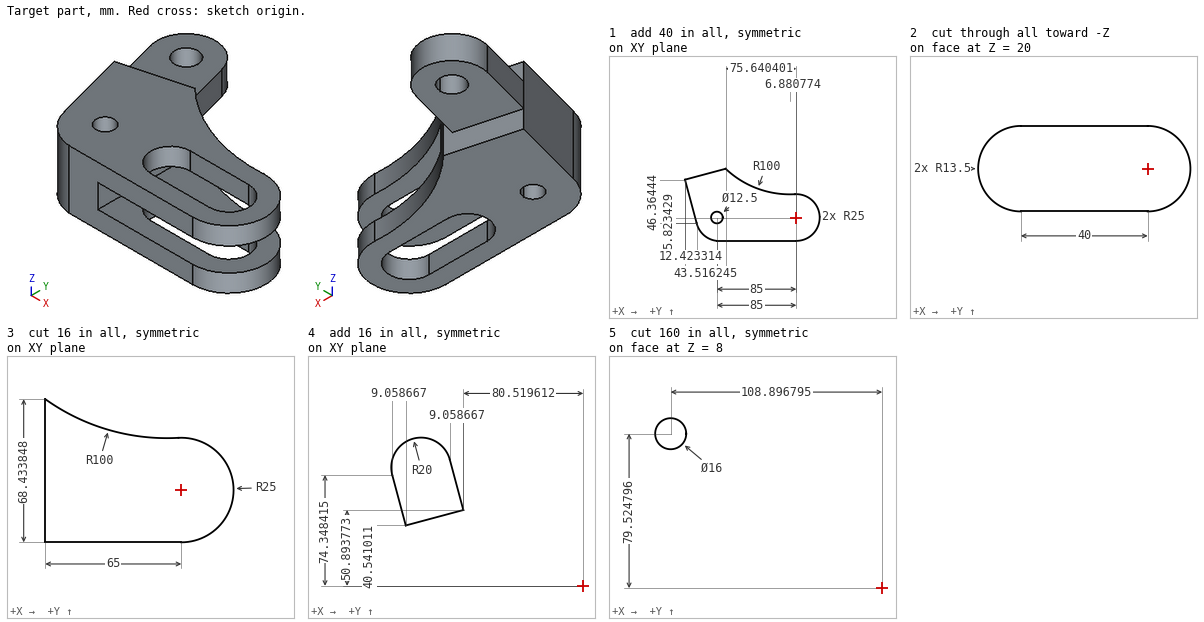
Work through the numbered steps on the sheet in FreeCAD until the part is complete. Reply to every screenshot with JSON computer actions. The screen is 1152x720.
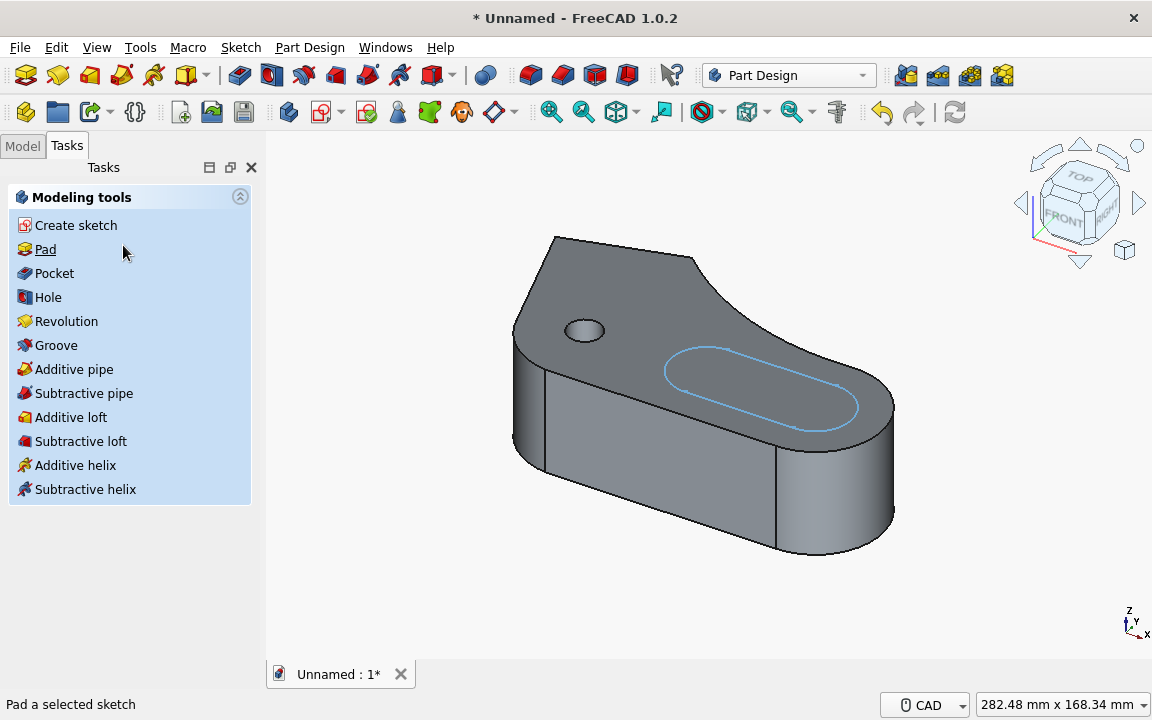
{"action": "left_click", "coordinate": [240, 76]}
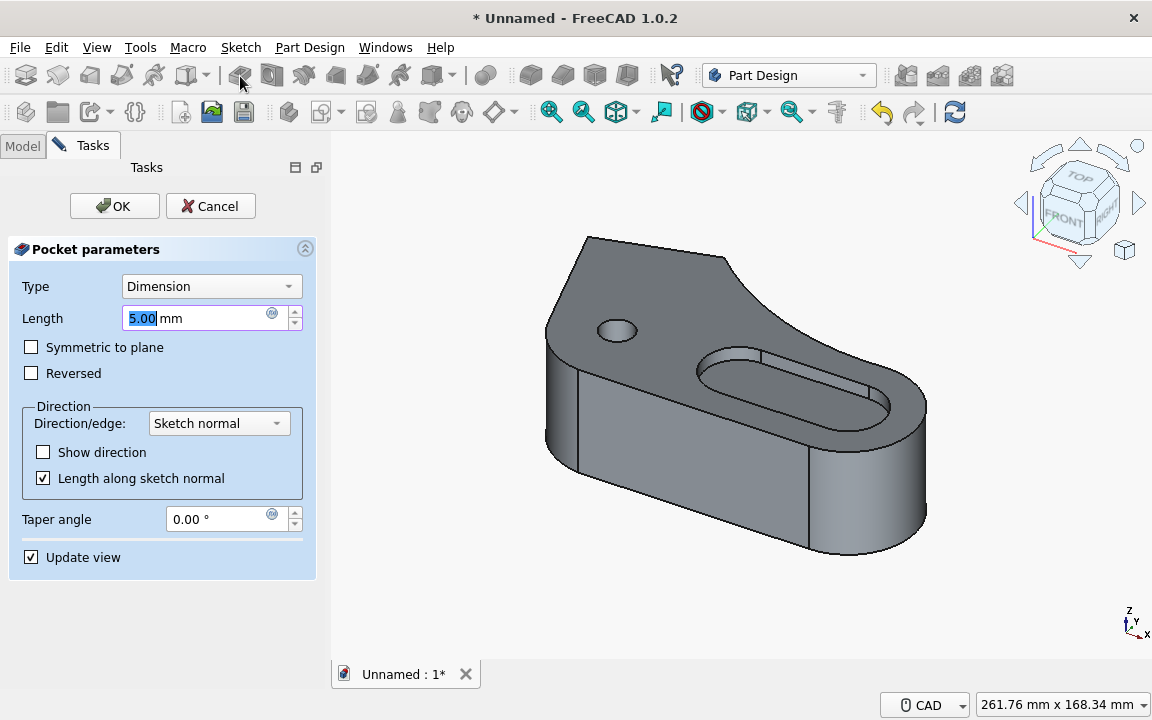
{"action": "left_click", "coordinate": [212, 286]}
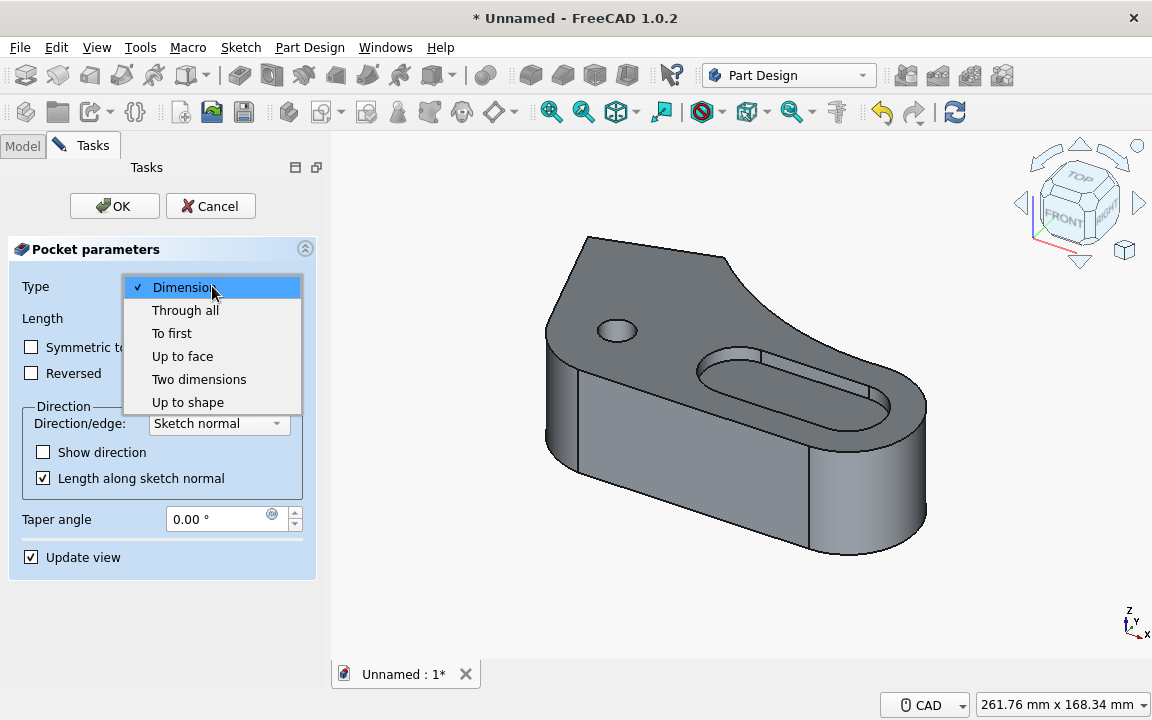
{"action": "left_click", "coordinate": [212, 310]}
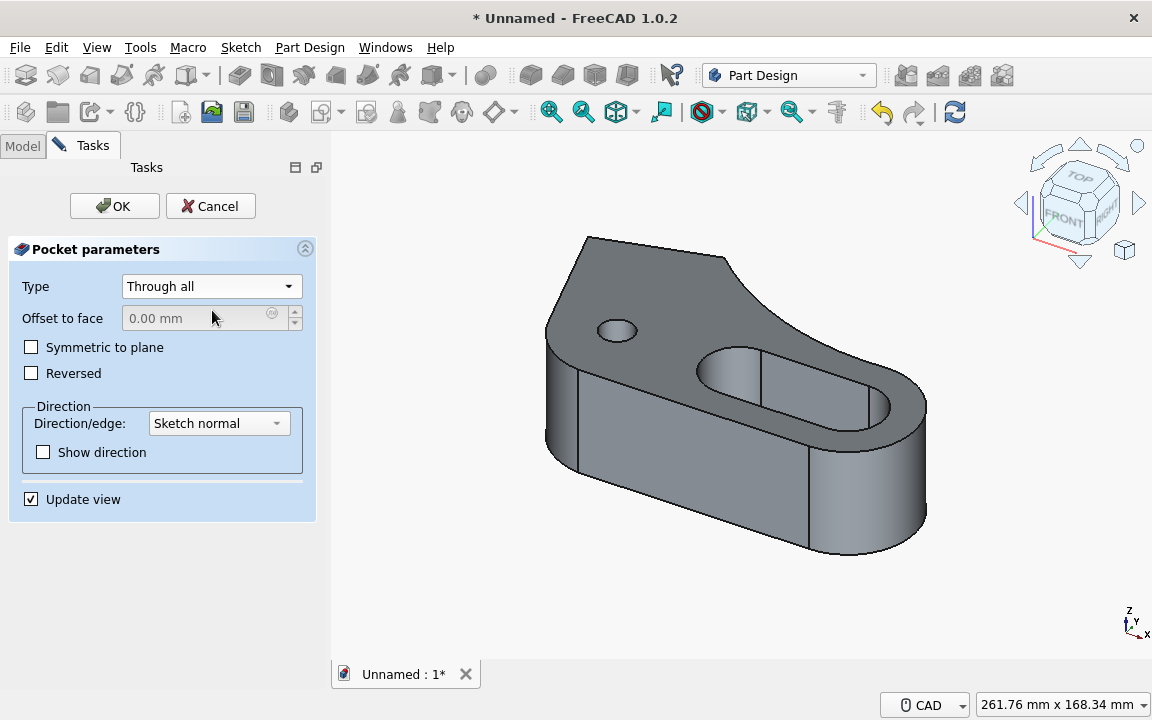
{"action": "left_click", "coordinate": [115, 206]}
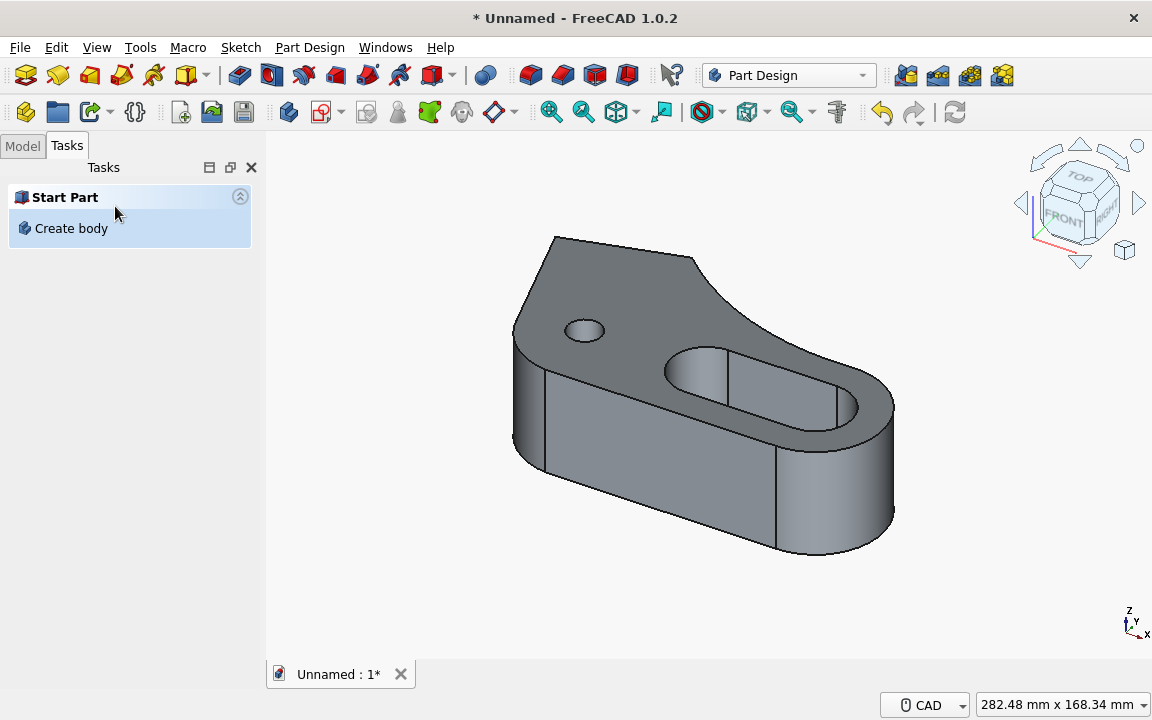
{"action": "left_click", "coordinate": [322, 112]}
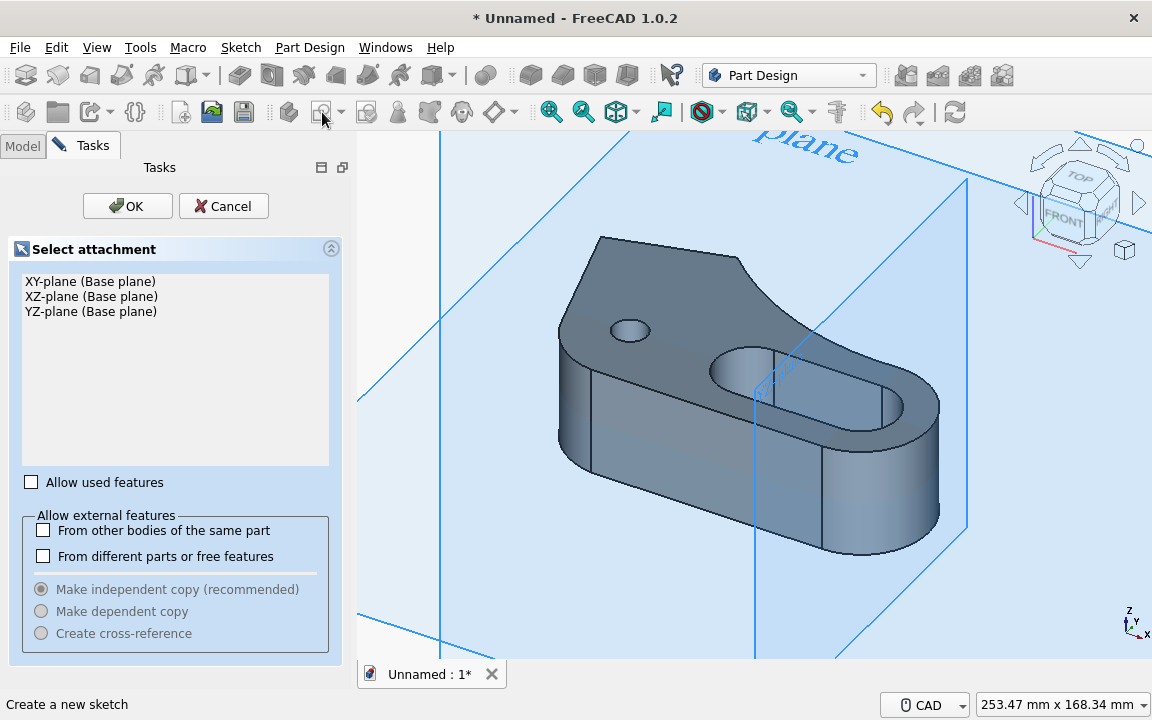
{"action": "left_click", "coordinate": [82, 282]}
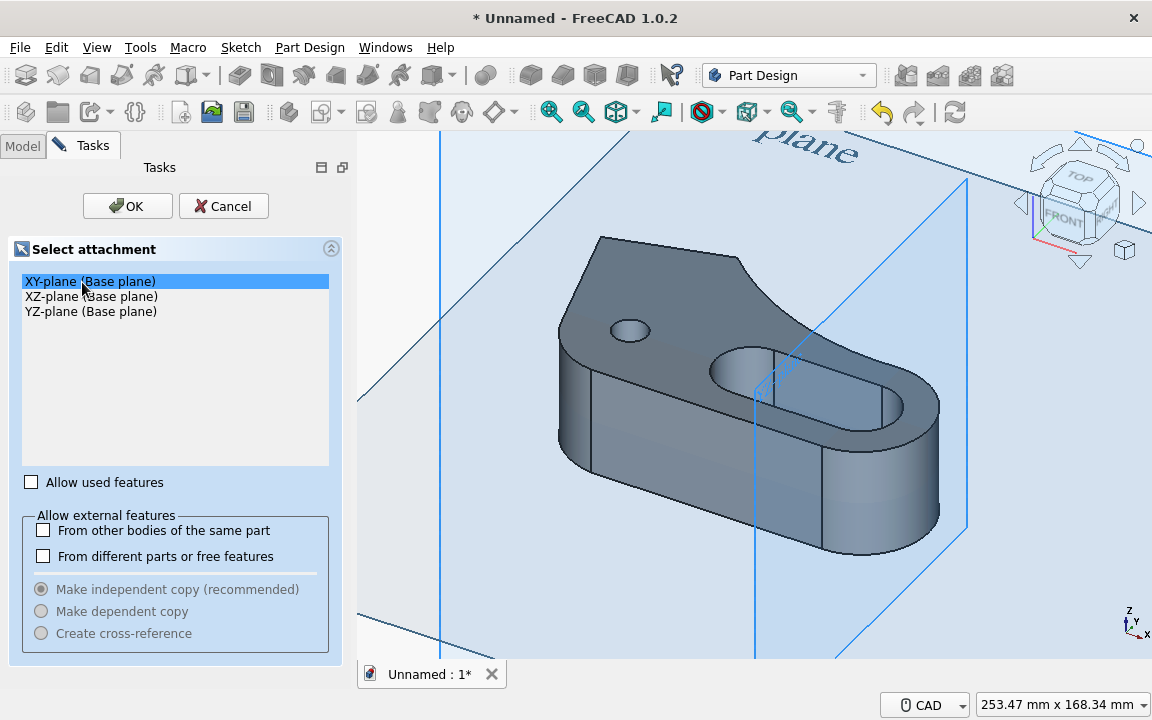
{"action": "left_click", "coordinate": [128, 206]}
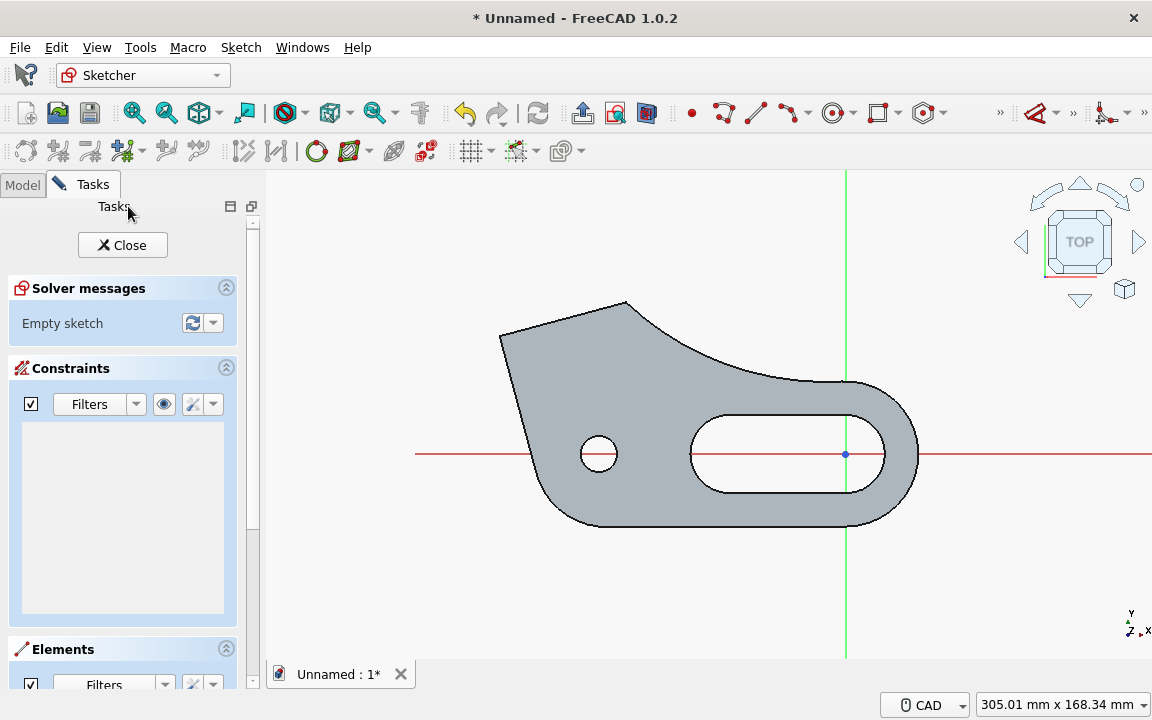
{"action": "left_click", "coordinate": [648, 114]}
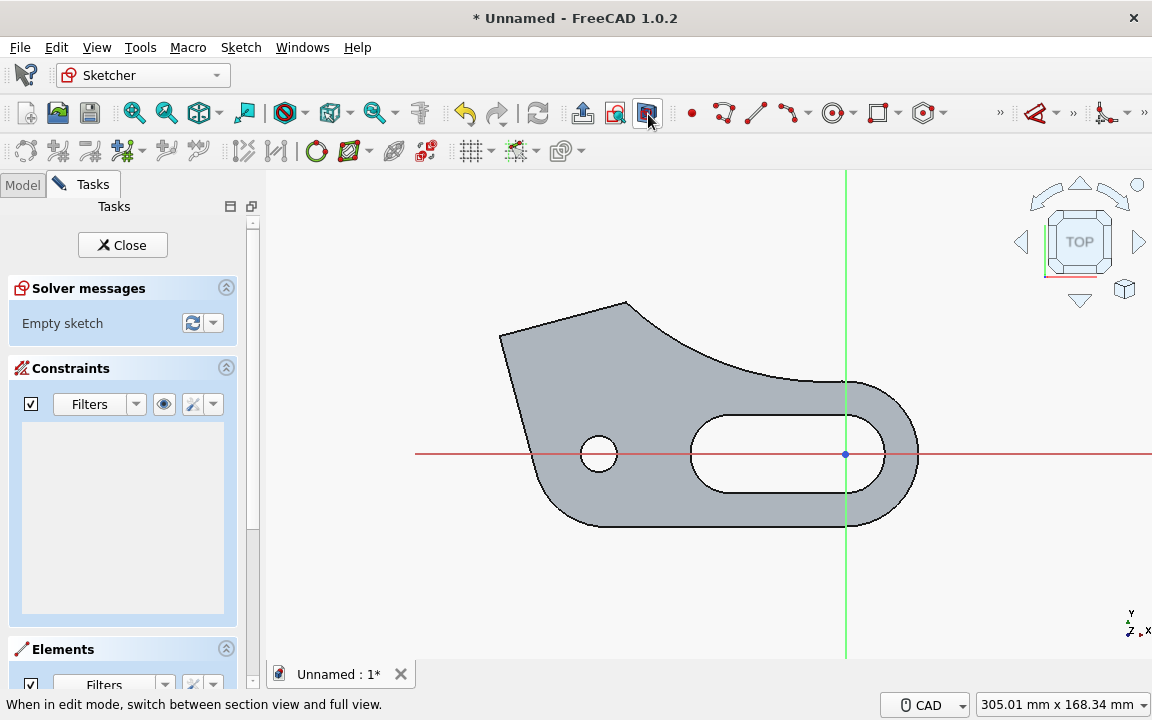
{"action": "scroll", "coordinate": [987, 453], "scroll_direction": "up", "scroll_amount": 2}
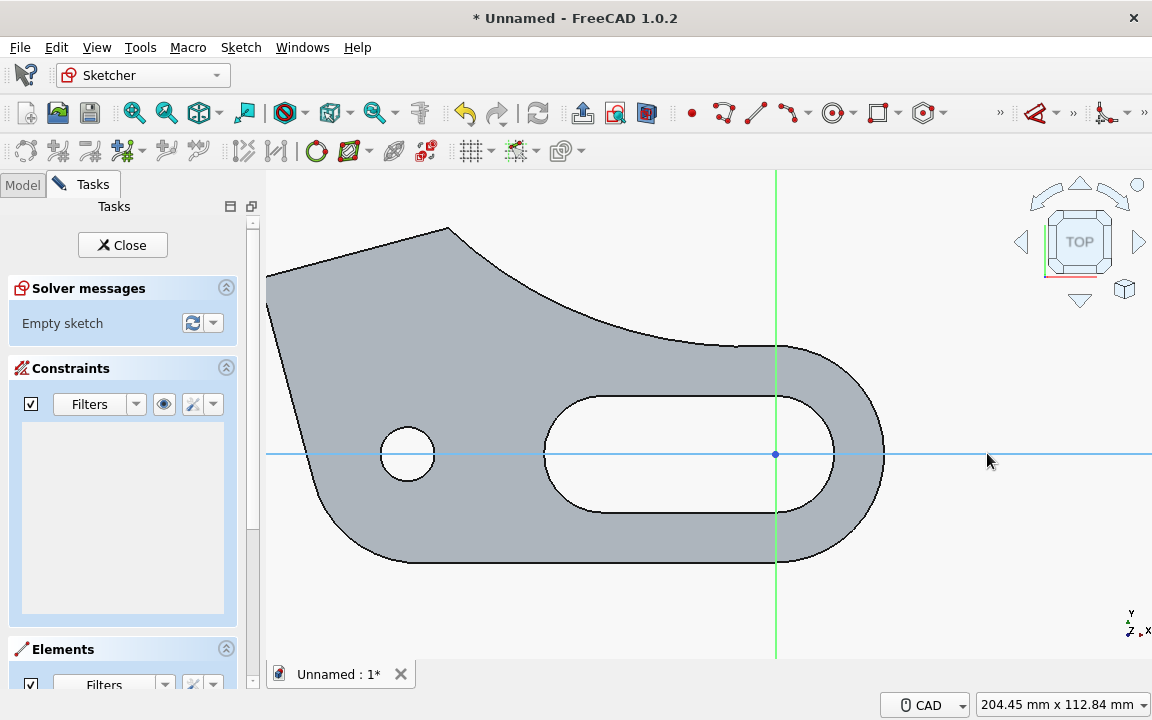
{"action": "left_click", "coordinate": [724, 114]}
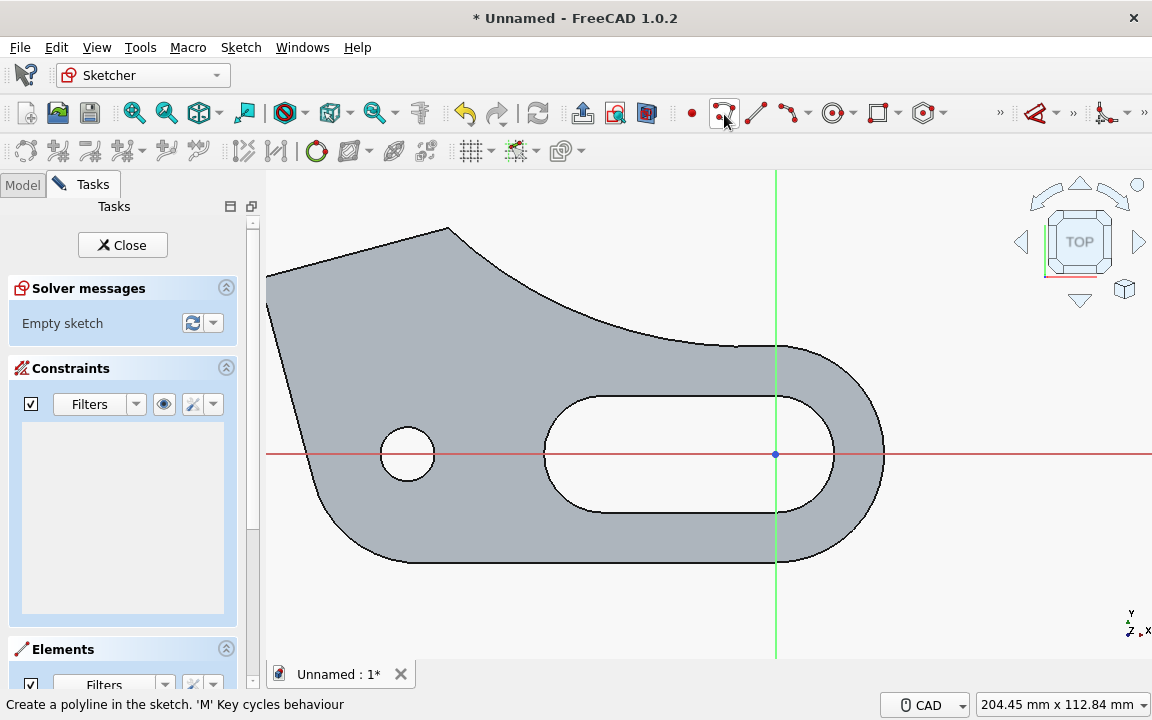
{"action": "left_click", "coordinate": [494, 266]}
{"action": "left_click", "coordinate": [494, 563]}
{"action": "left_click", "coordinate": [776, 563]}
{"action": "right_click", "coordinate": [776, 563]}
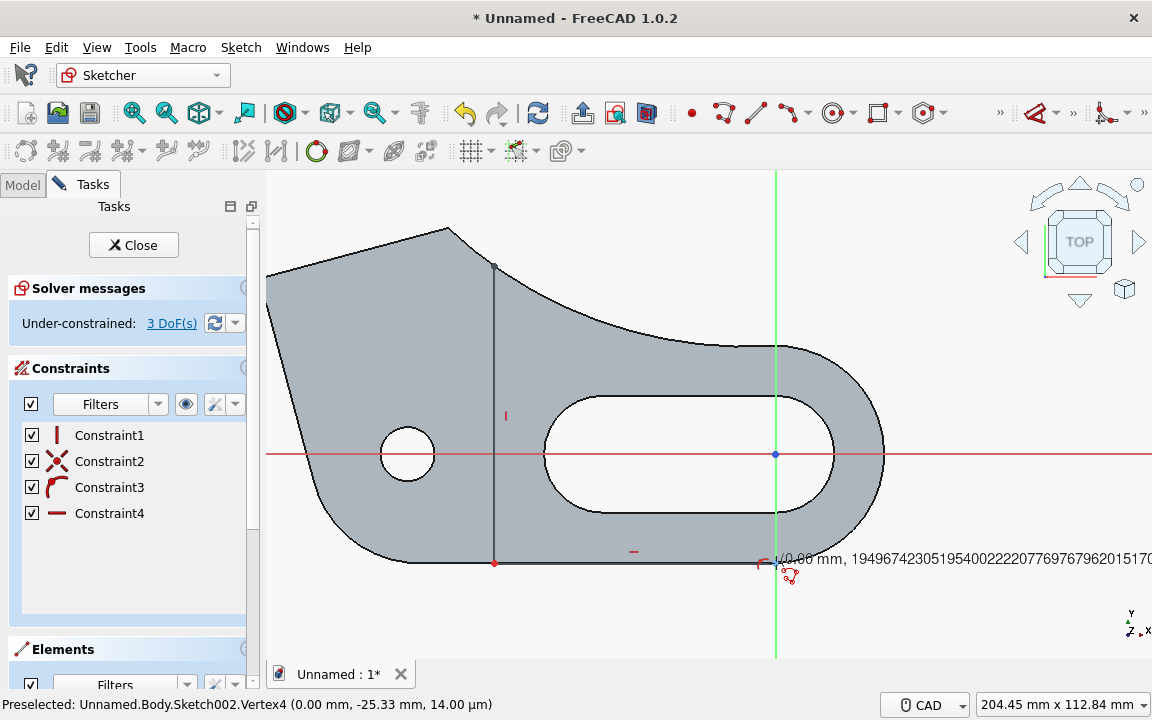
{"action": "left_click", "coordinate": [788, 114]}